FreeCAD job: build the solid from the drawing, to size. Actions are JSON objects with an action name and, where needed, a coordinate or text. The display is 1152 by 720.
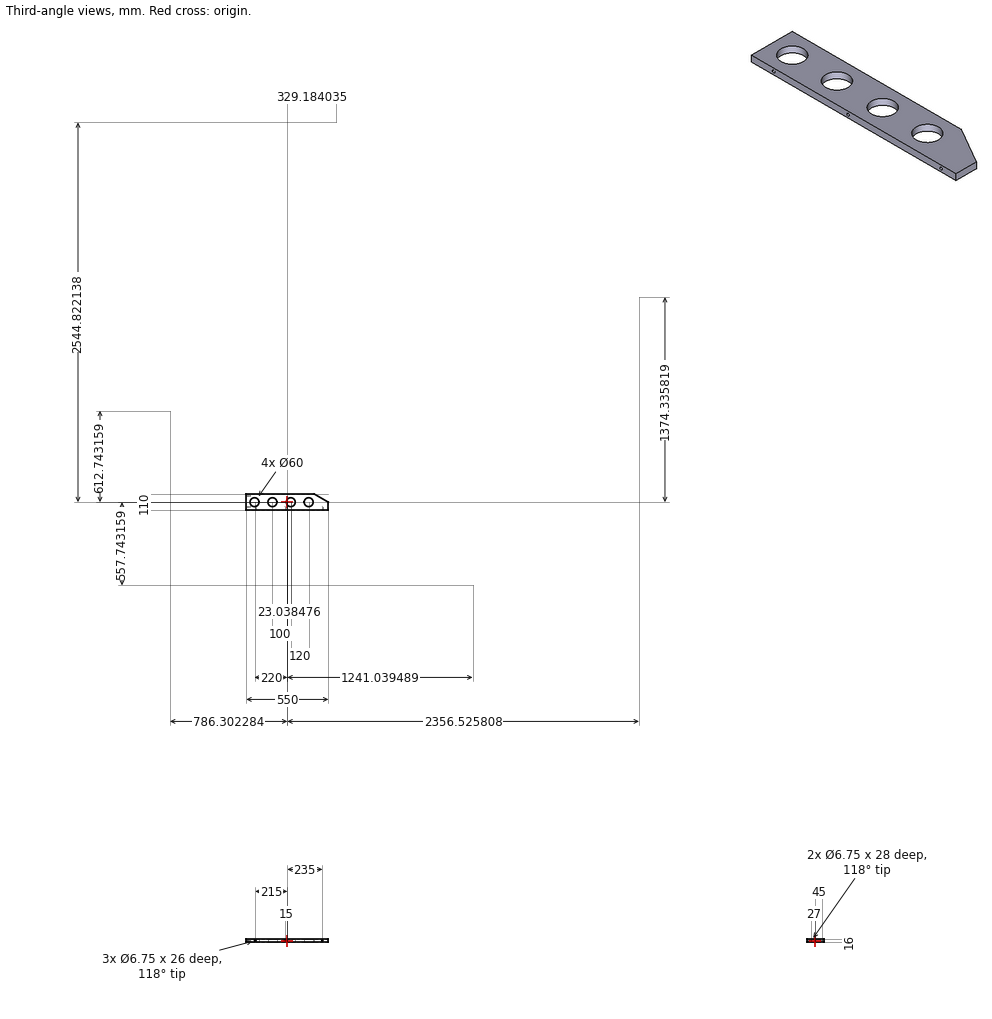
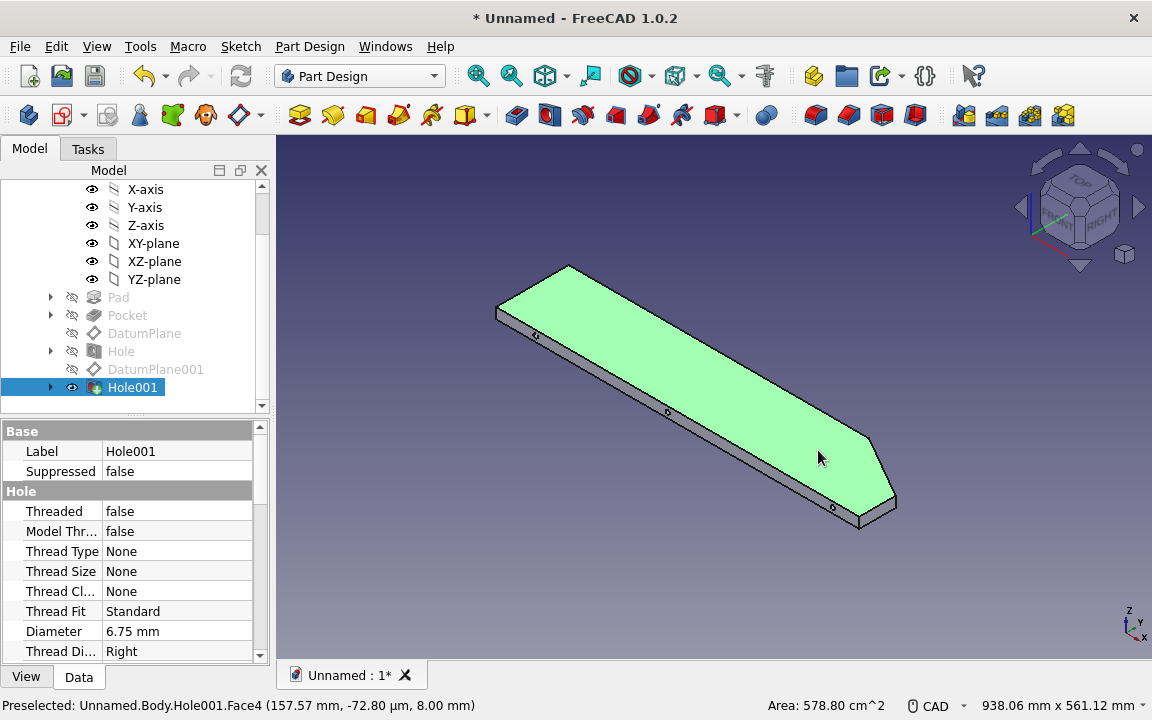
{"action": "left_click", "coordinate": [62, 116]}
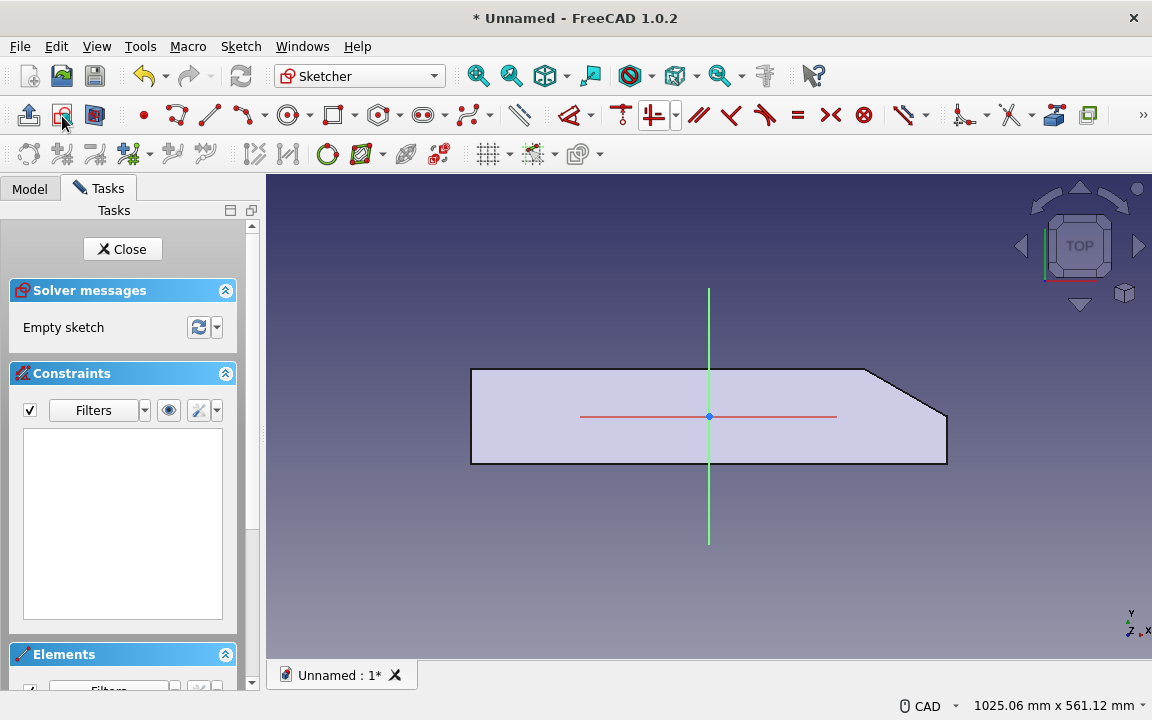
{"action": "key", "text": "g c"}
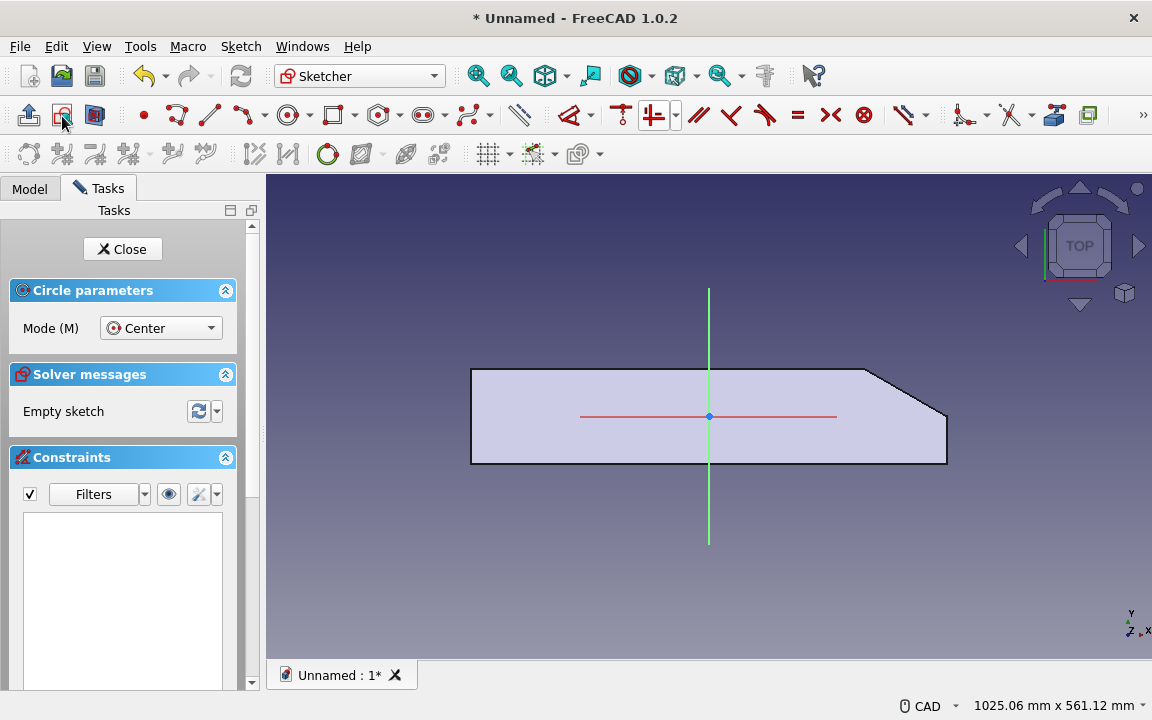
{"action": "left_click", "coordinate": [519, 416]}
{"action": "mouse_move", "coordinate": [537, 398]}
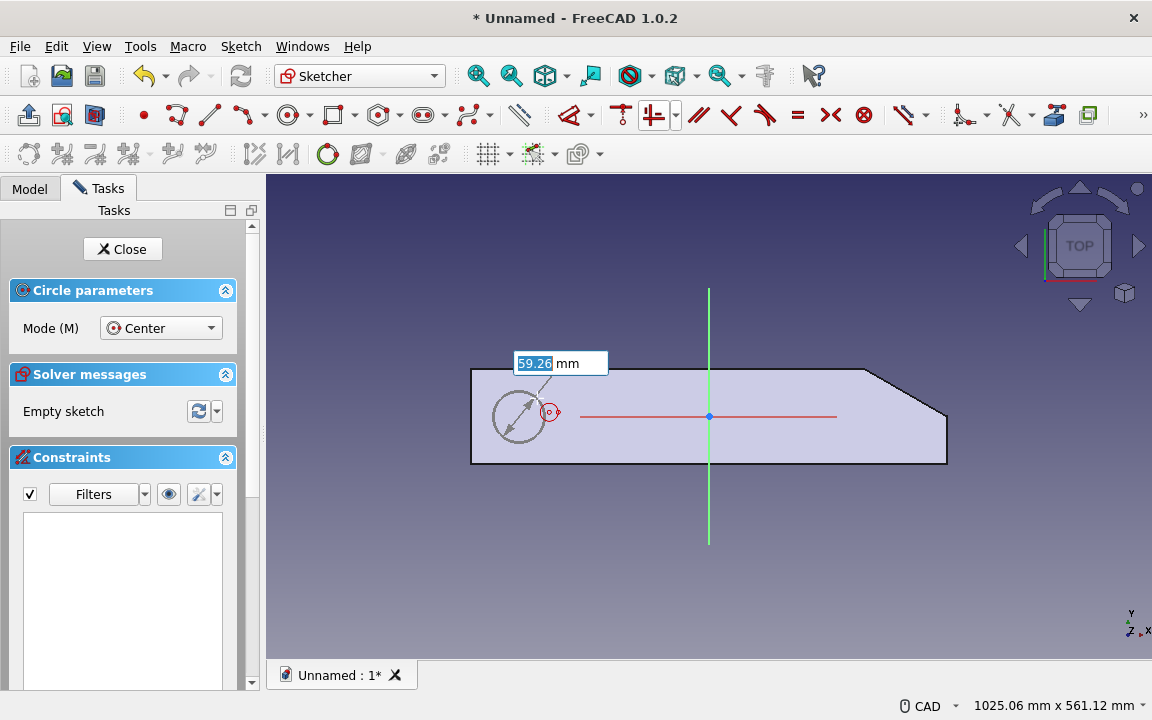
{"action": "type", "text": "60"}
{"action": "key", "text": "Return"}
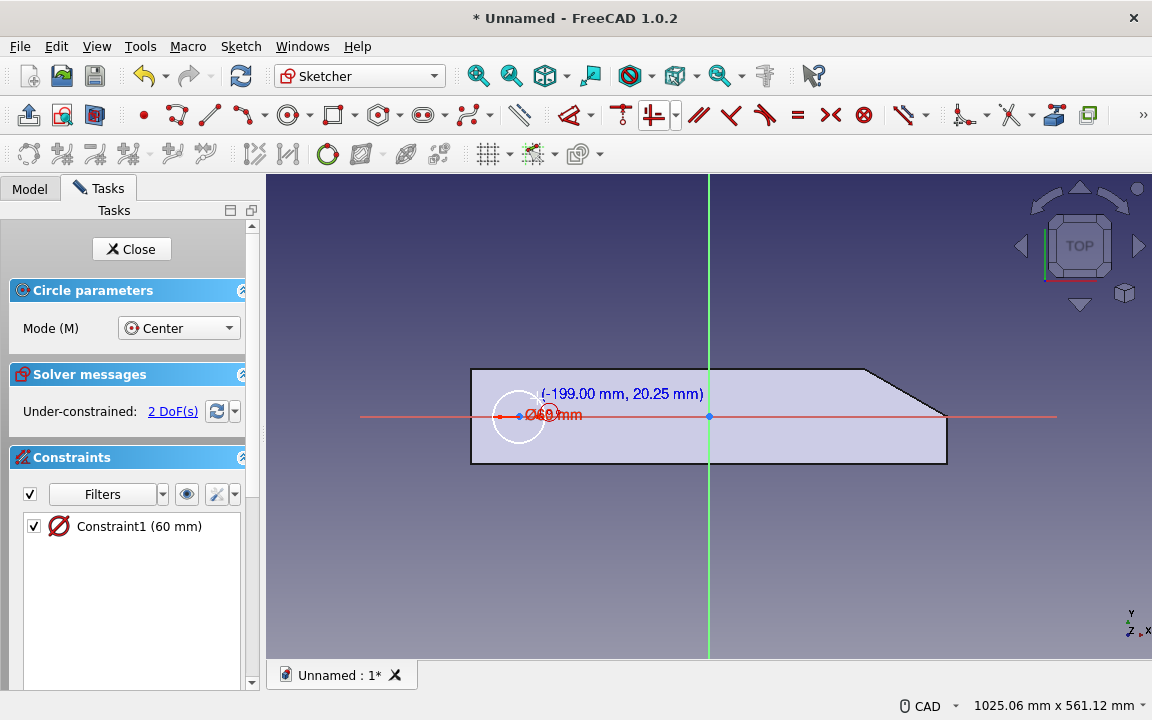
{"action": "left_click", "coordinate": [623, 416]}
{"action": "mouse_move", "coordinate": [641, 398]}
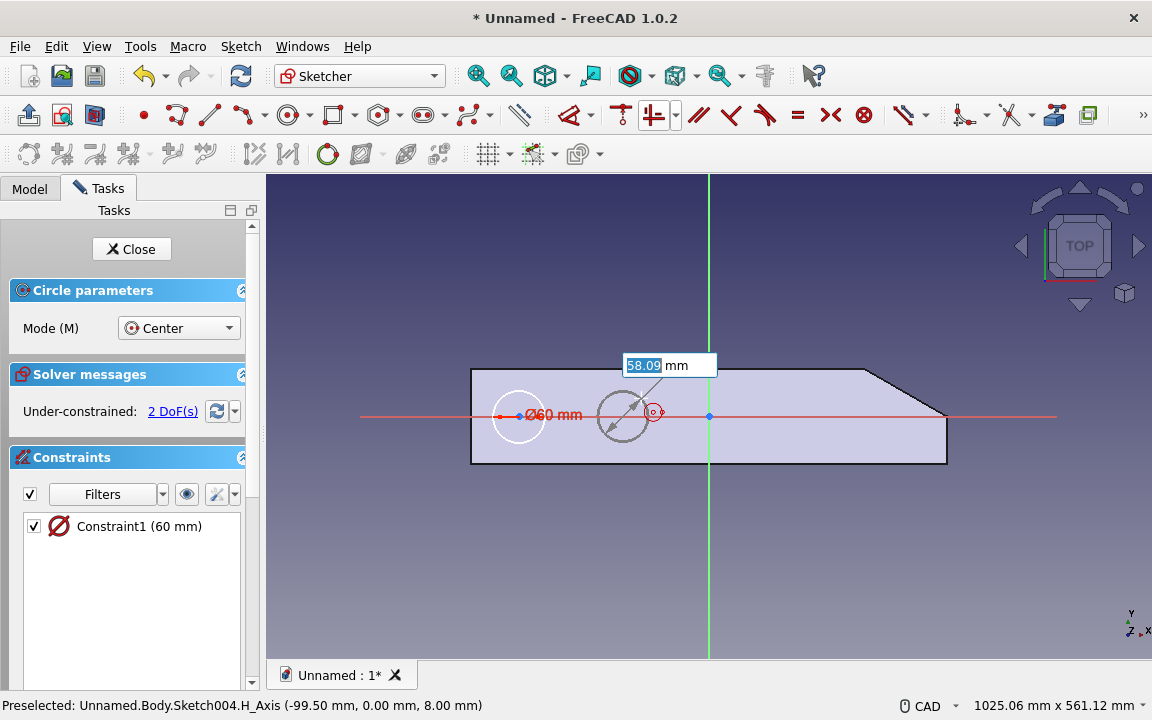
{"action": "type", "text": "60"}
{"action": "key", "text": "Return"}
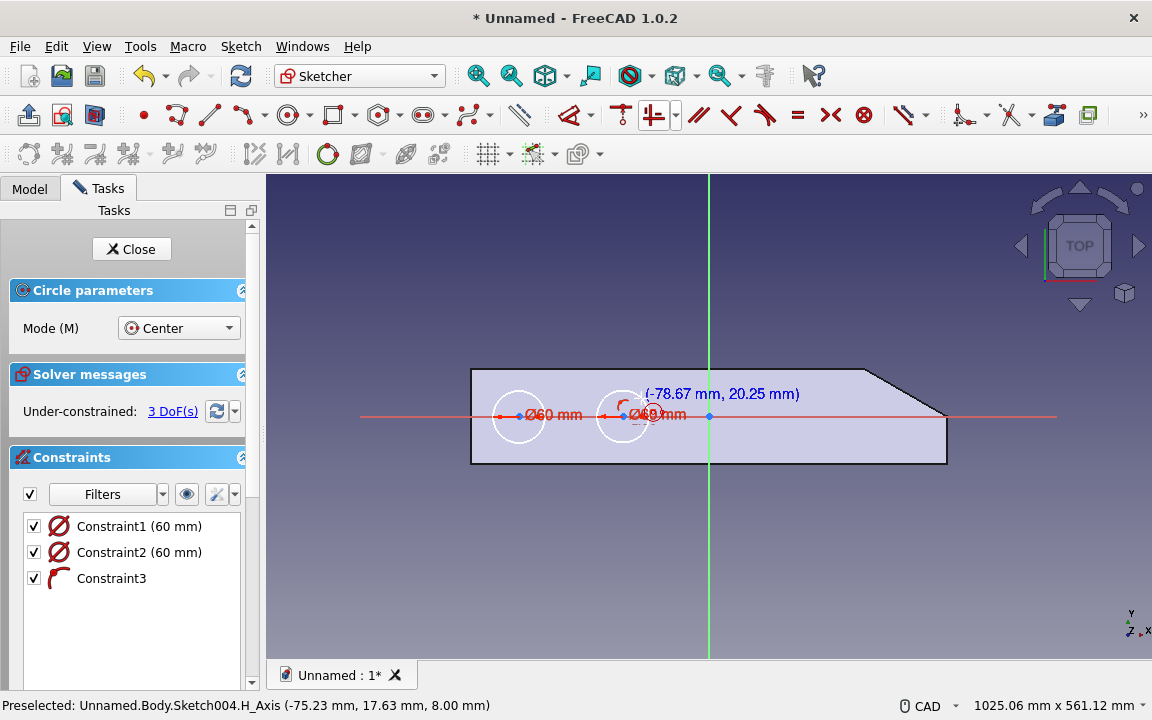
{"action": "left_click", "coordinate": [729, 416]}
{"action": "mouse_move", "coordinate": [747, 398]}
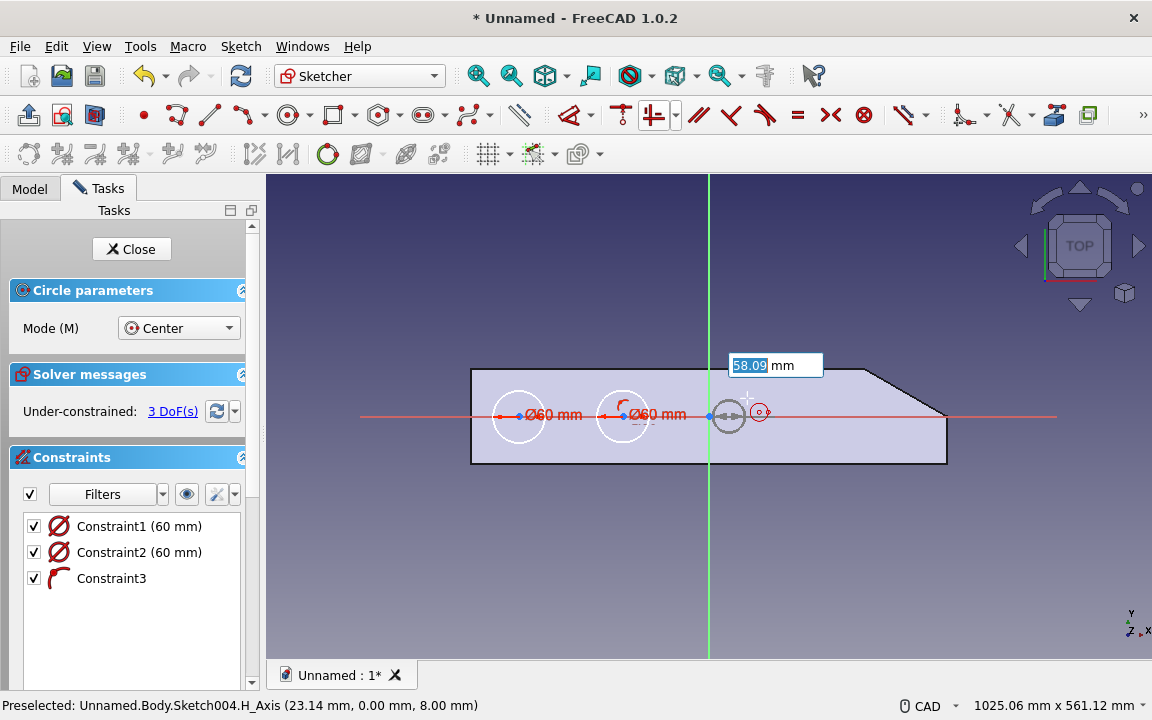
{"action": "type", "text": "60"}
{"action": "key", "text": "Return"}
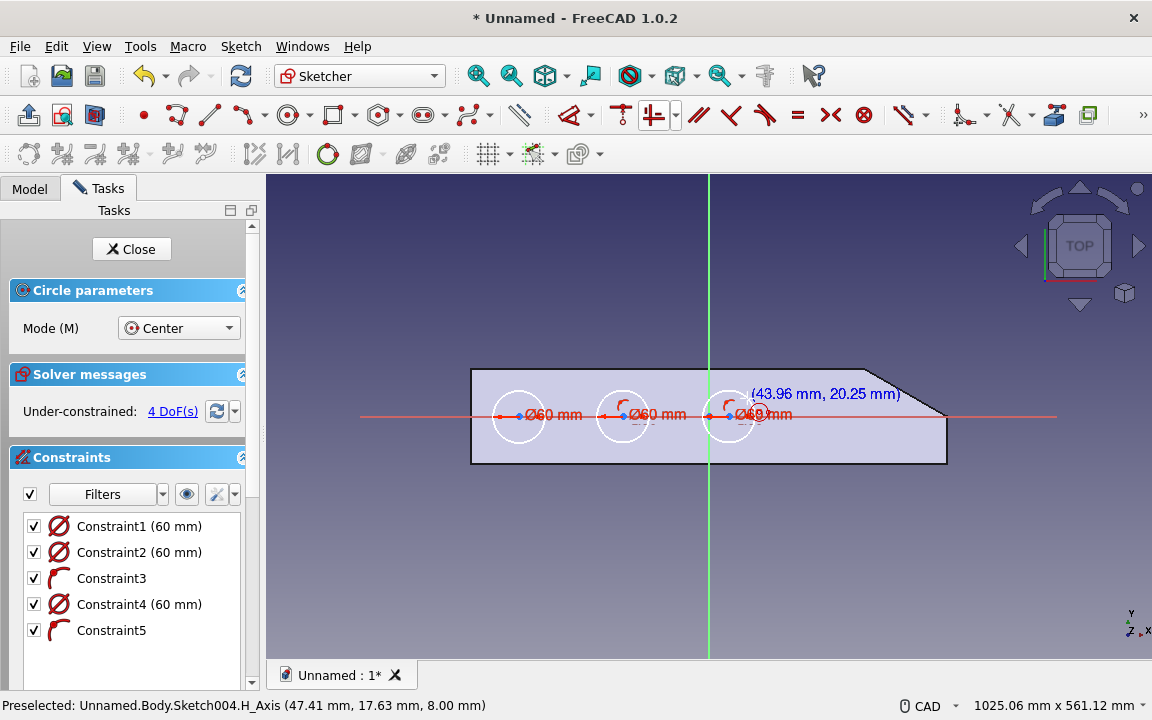
{"action": "left_click", "coordinate": [833, 416]}
{"action": "mouse_move", "coordinate": [851, 398]}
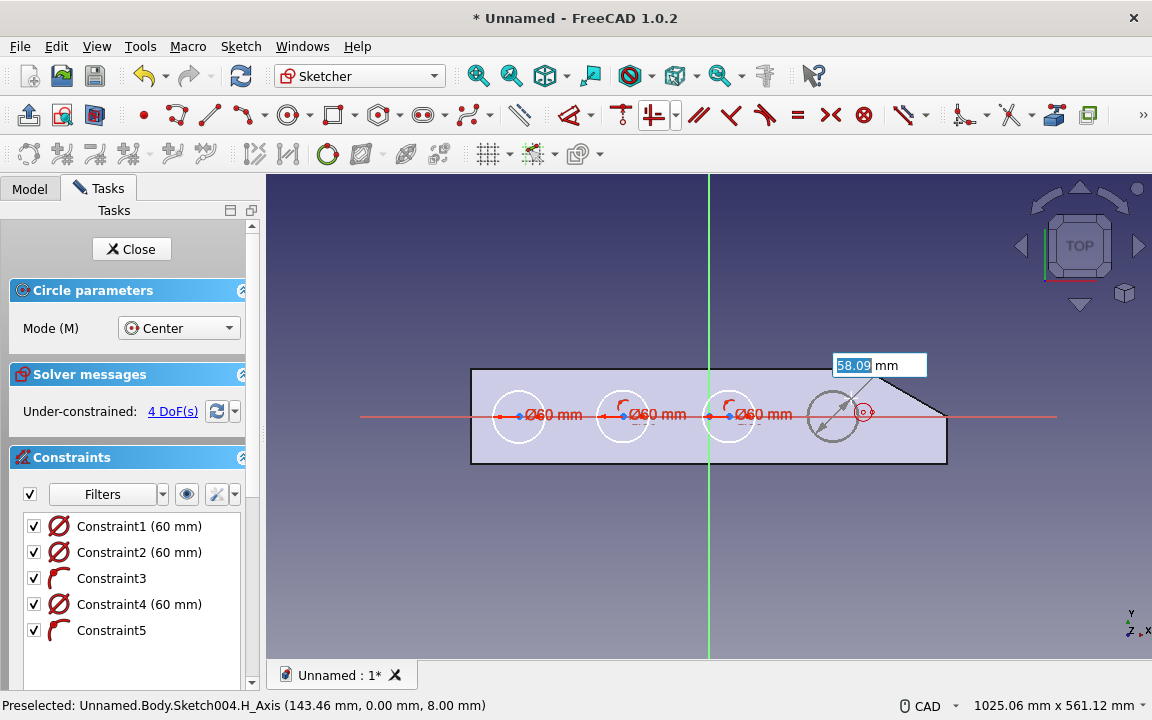
{"action": "type", "text": "60"}
{"action": "key", "text": "Return"}
{"action": "key", "text": "Escape"}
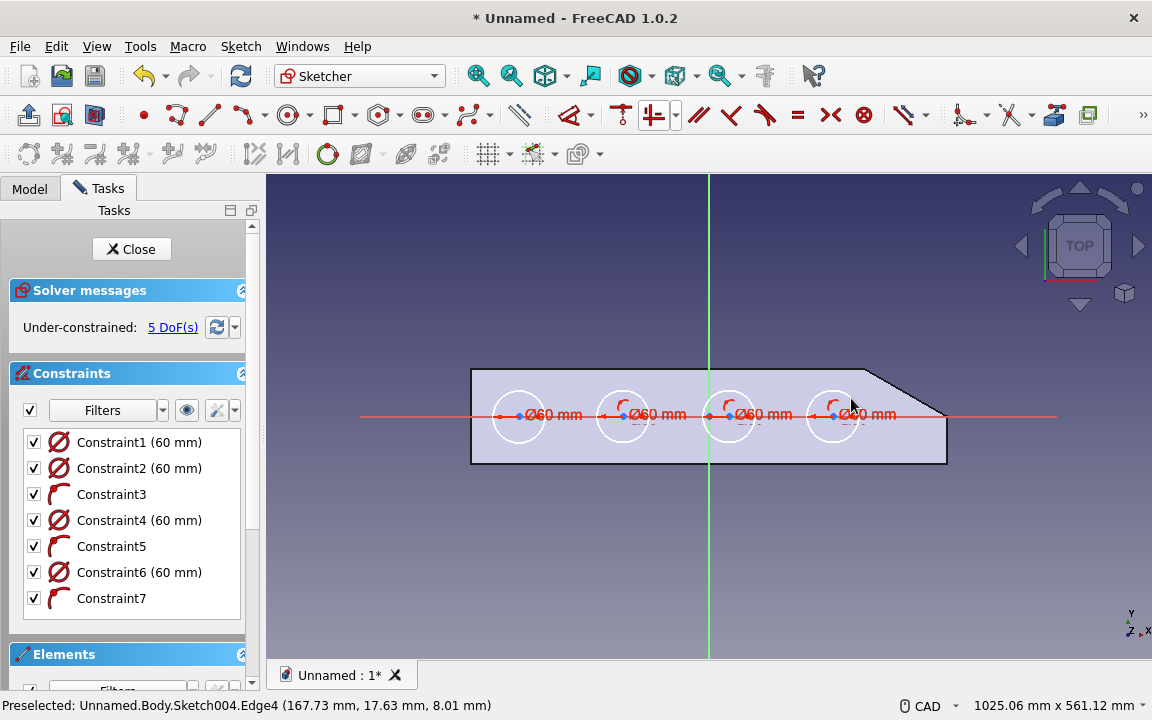
{"action": "left_click", "coordinate": [519, 417]}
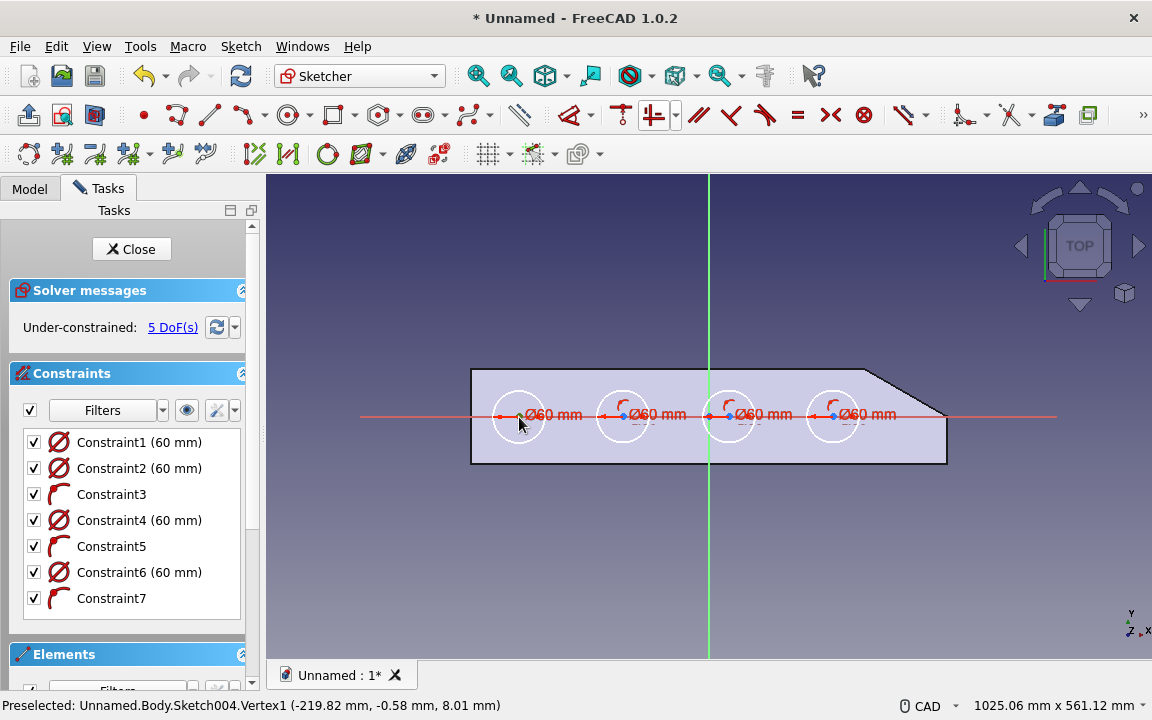
{"action": "left_click", "coordinate": [393, 416]}